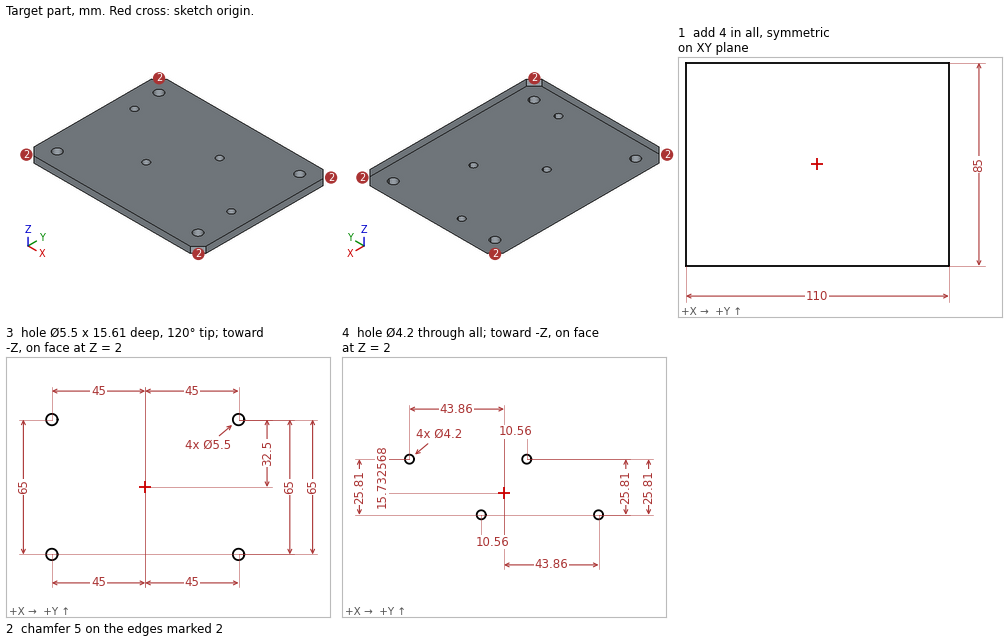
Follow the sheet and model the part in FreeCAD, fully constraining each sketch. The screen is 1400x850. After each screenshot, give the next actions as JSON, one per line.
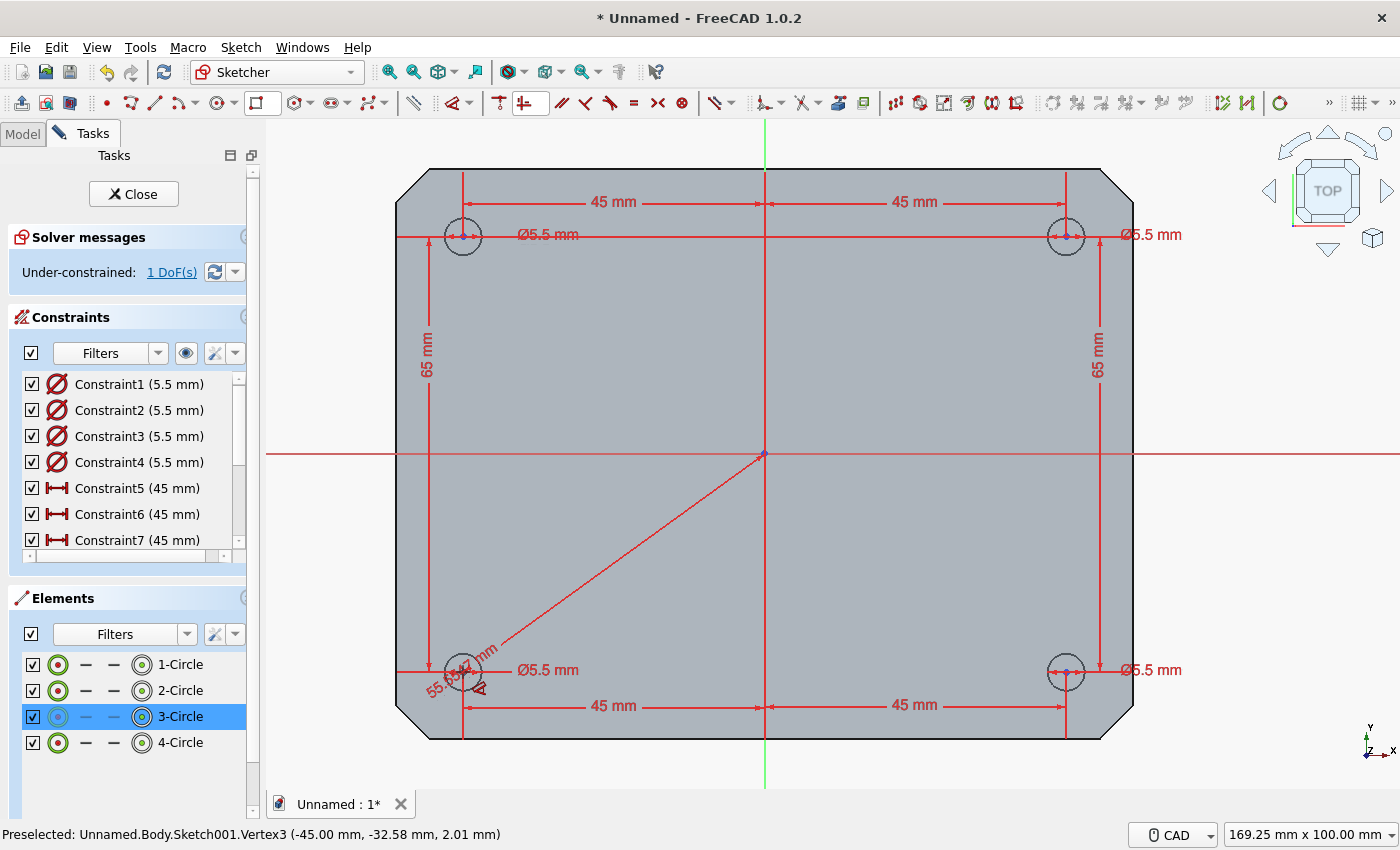
{"action": "left_click", "coordinate": [463, 237]}
{"action": "left_click", "coordinate": [429, 555]}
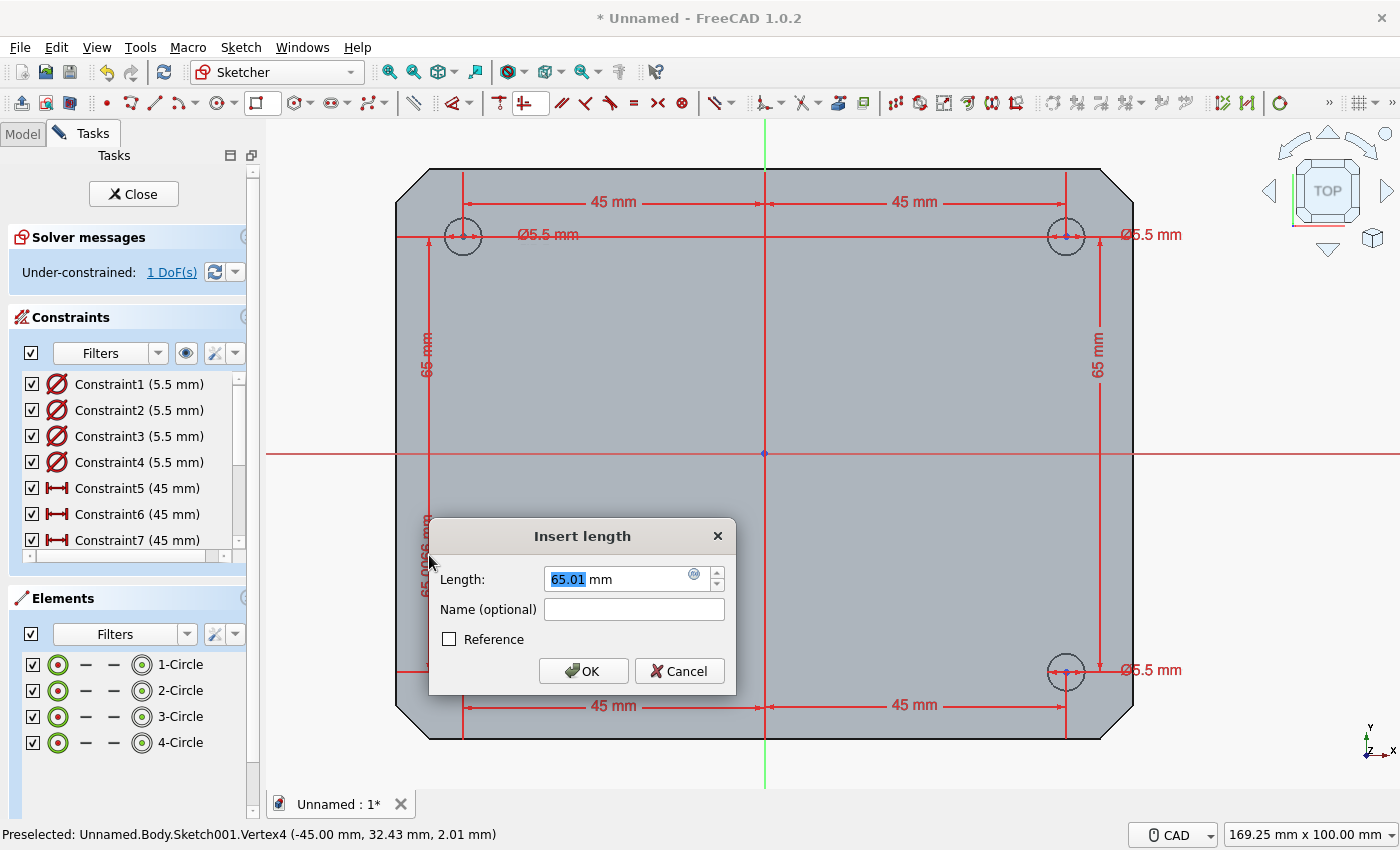
{"action": "type", "text": "65"}
{"action": "key", "text": "Return"}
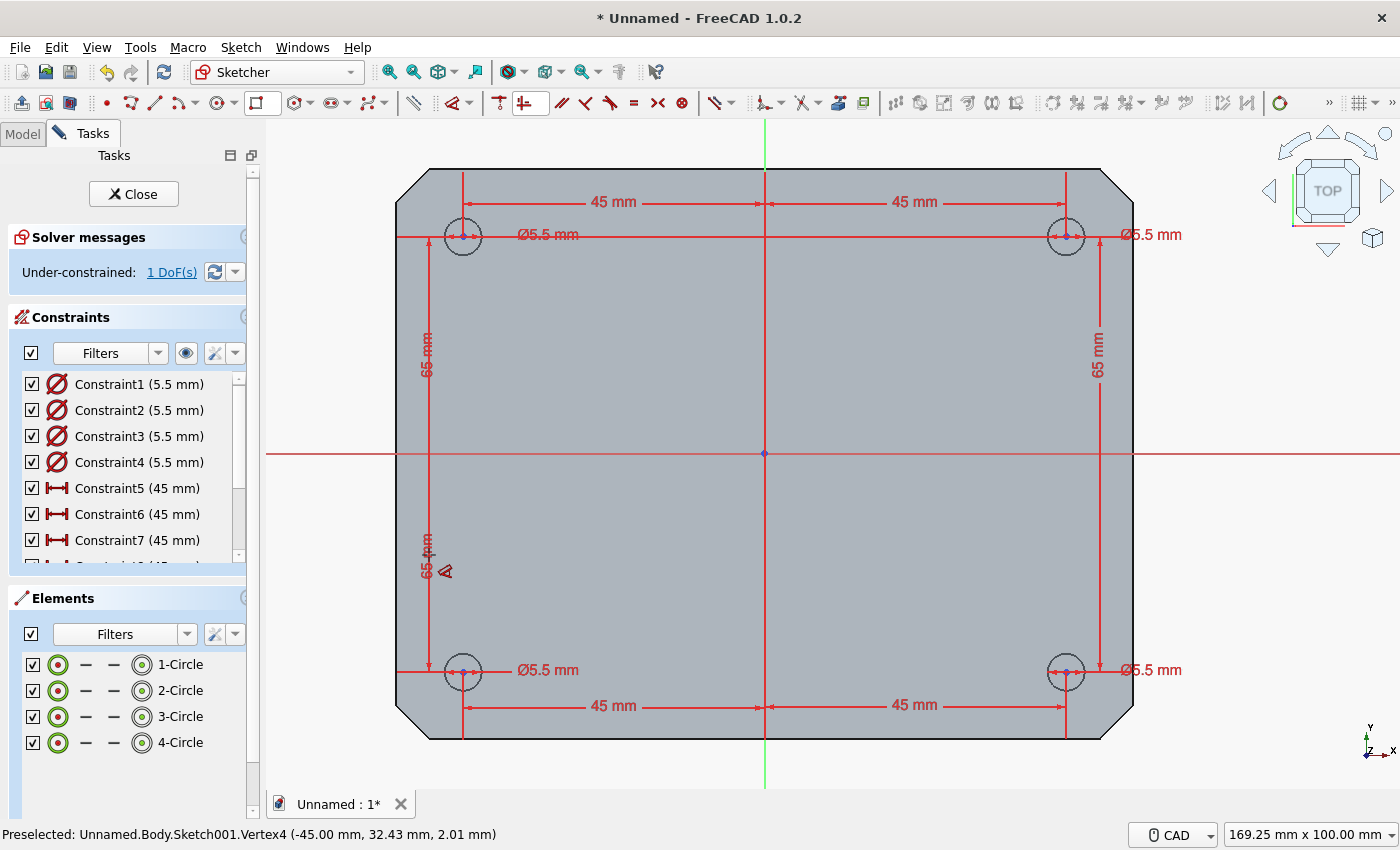
{"action": "left_click", "coordinate": [1066, 237]}
{"action": "left_click", "coordinate": [1100, 295]}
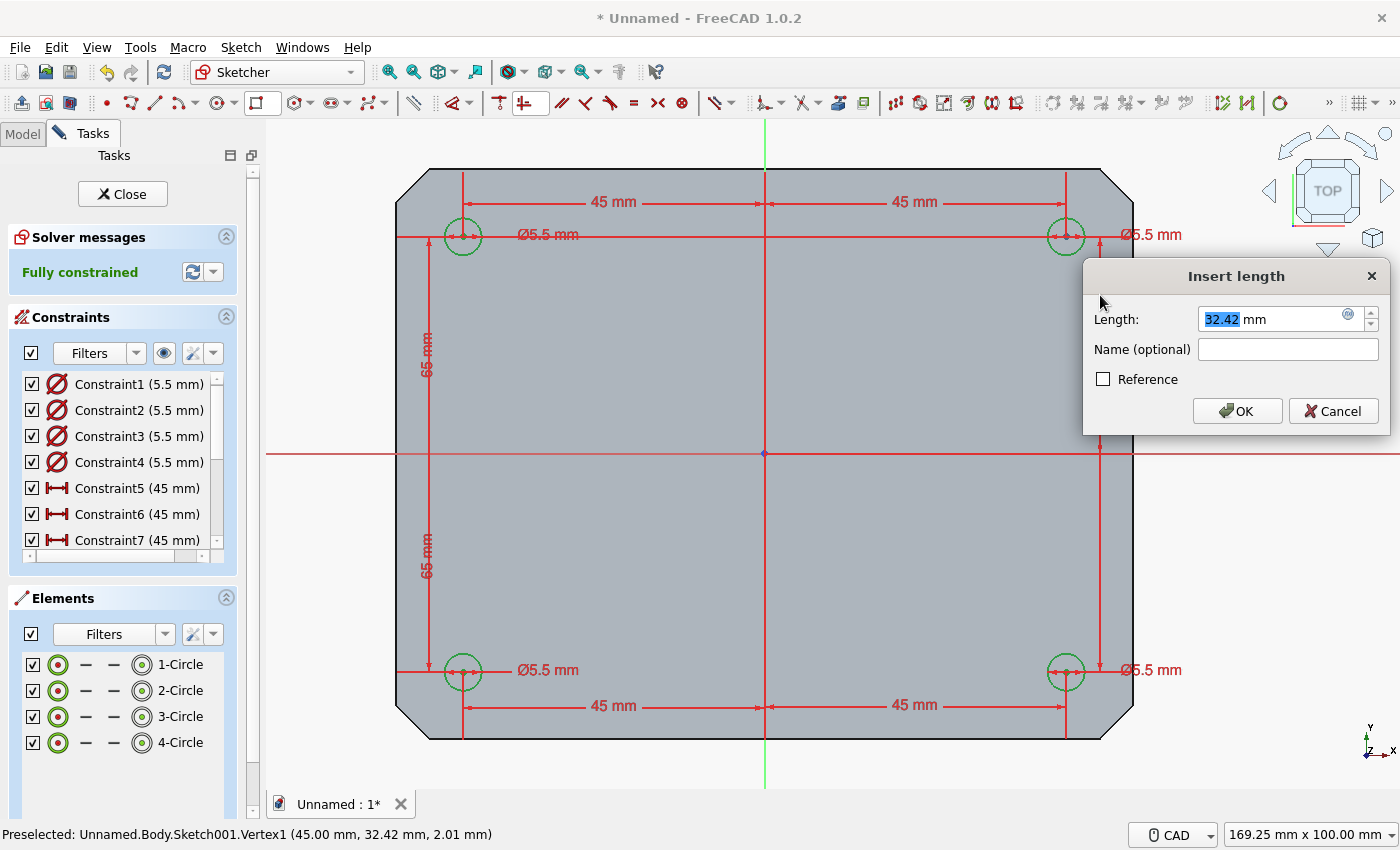
{"action": "type", "text": "32.5"}
{"action": "key", "text": "Return"}
{"action": "key", "text": "Escape"}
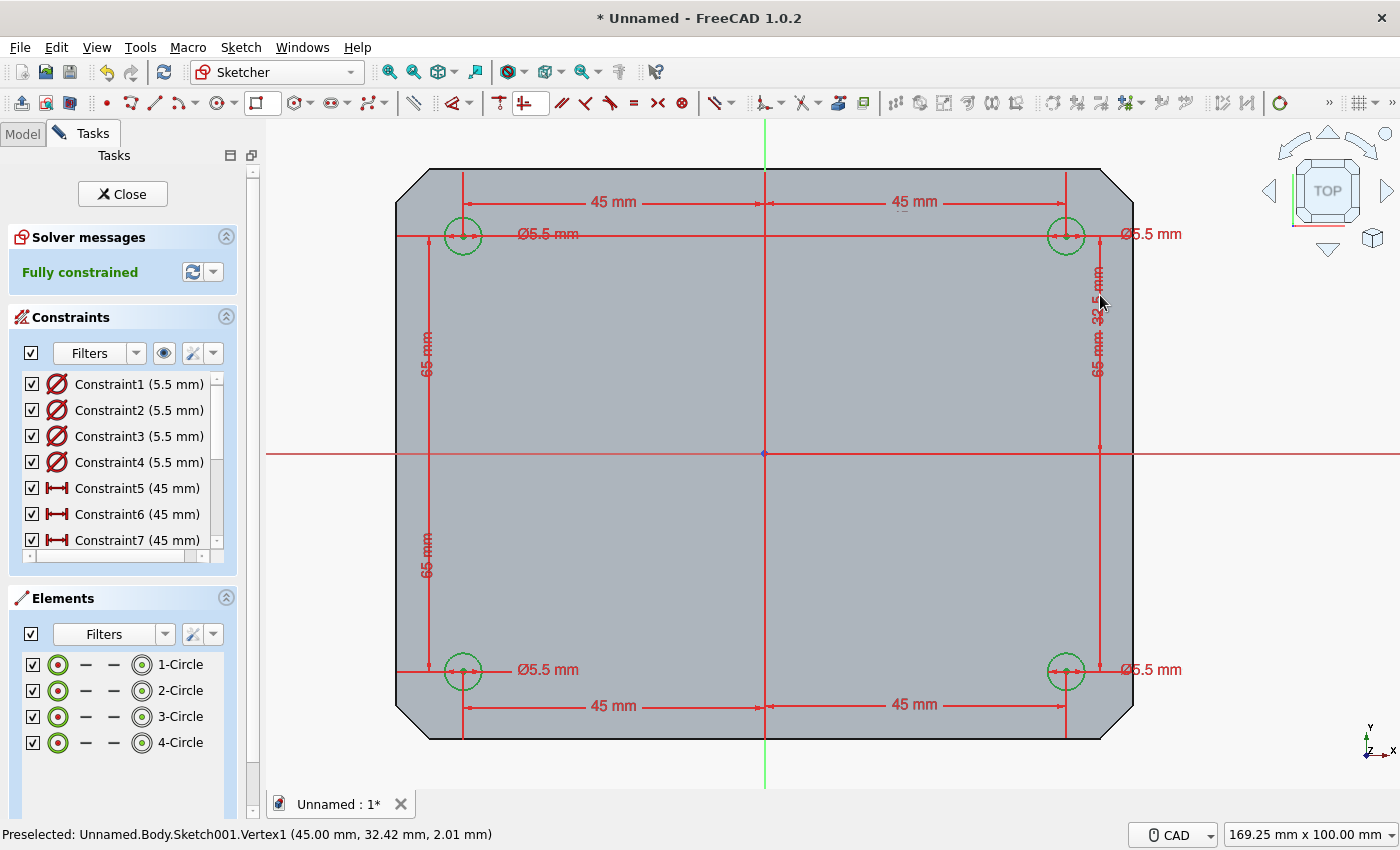
{"action": "left_click", "coordinate": [123, 194]}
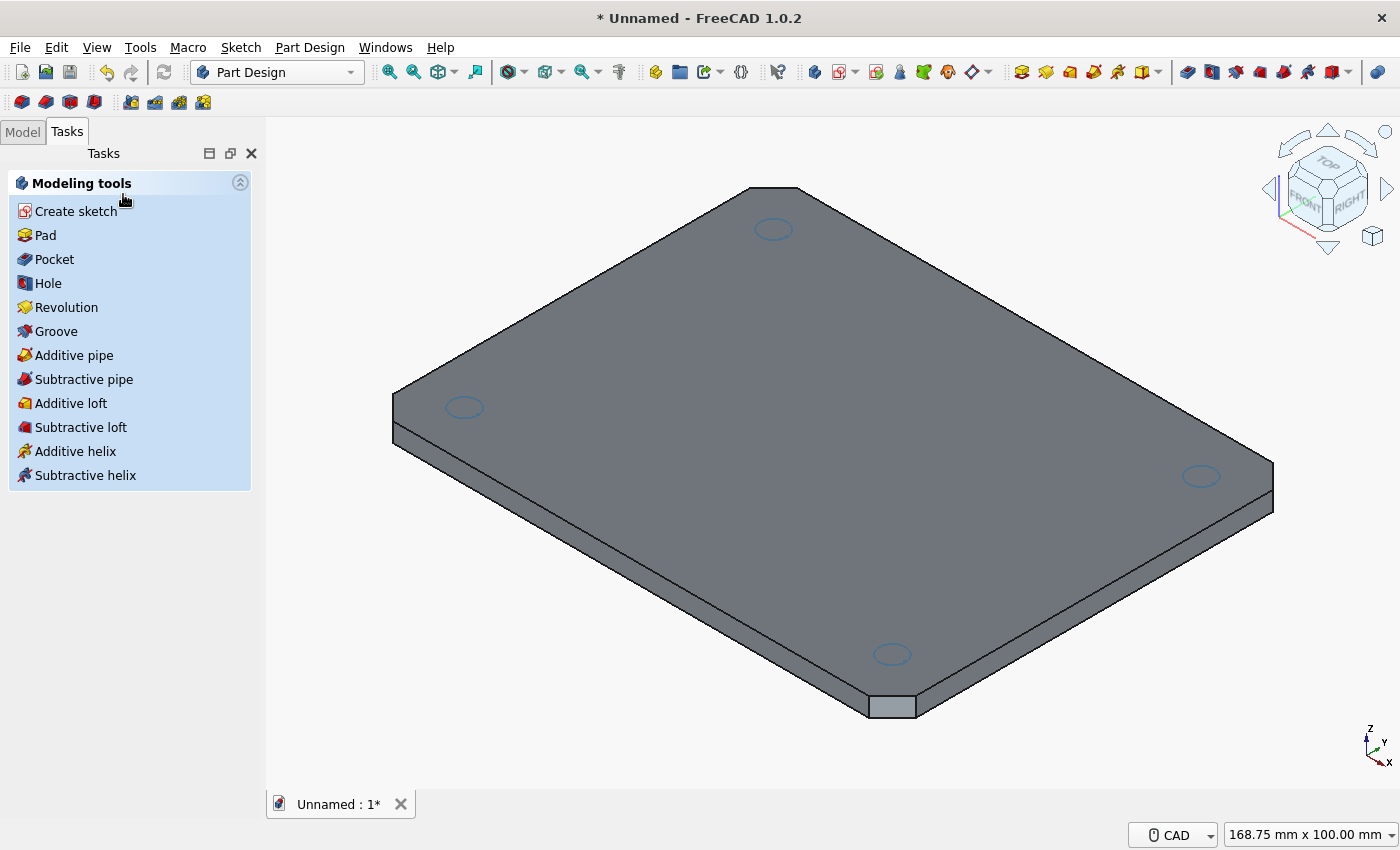
{"action": "left_click", "coordinate": [1212, 72]}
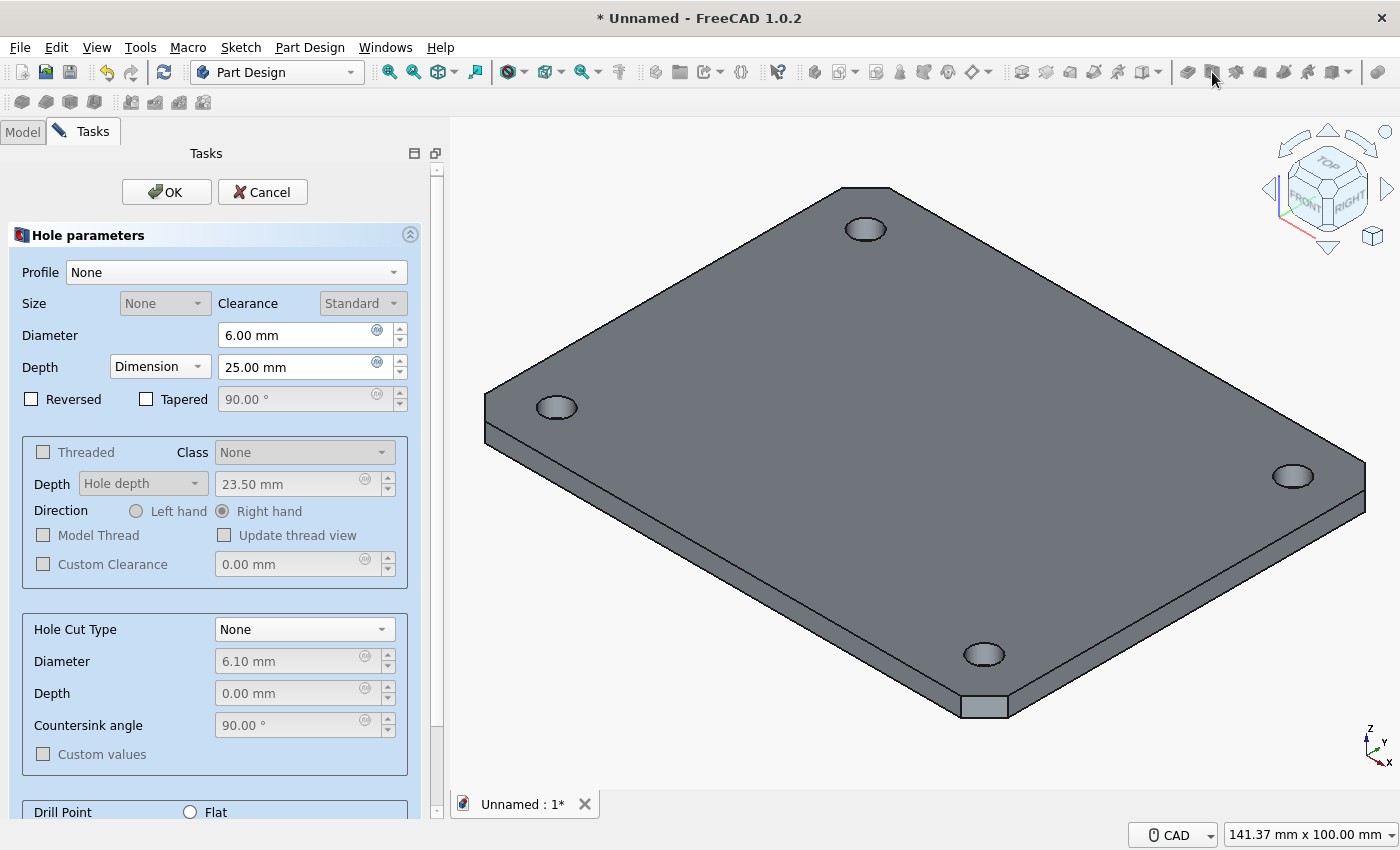
{"action": "triple_click", "coordinate": [305, 335]}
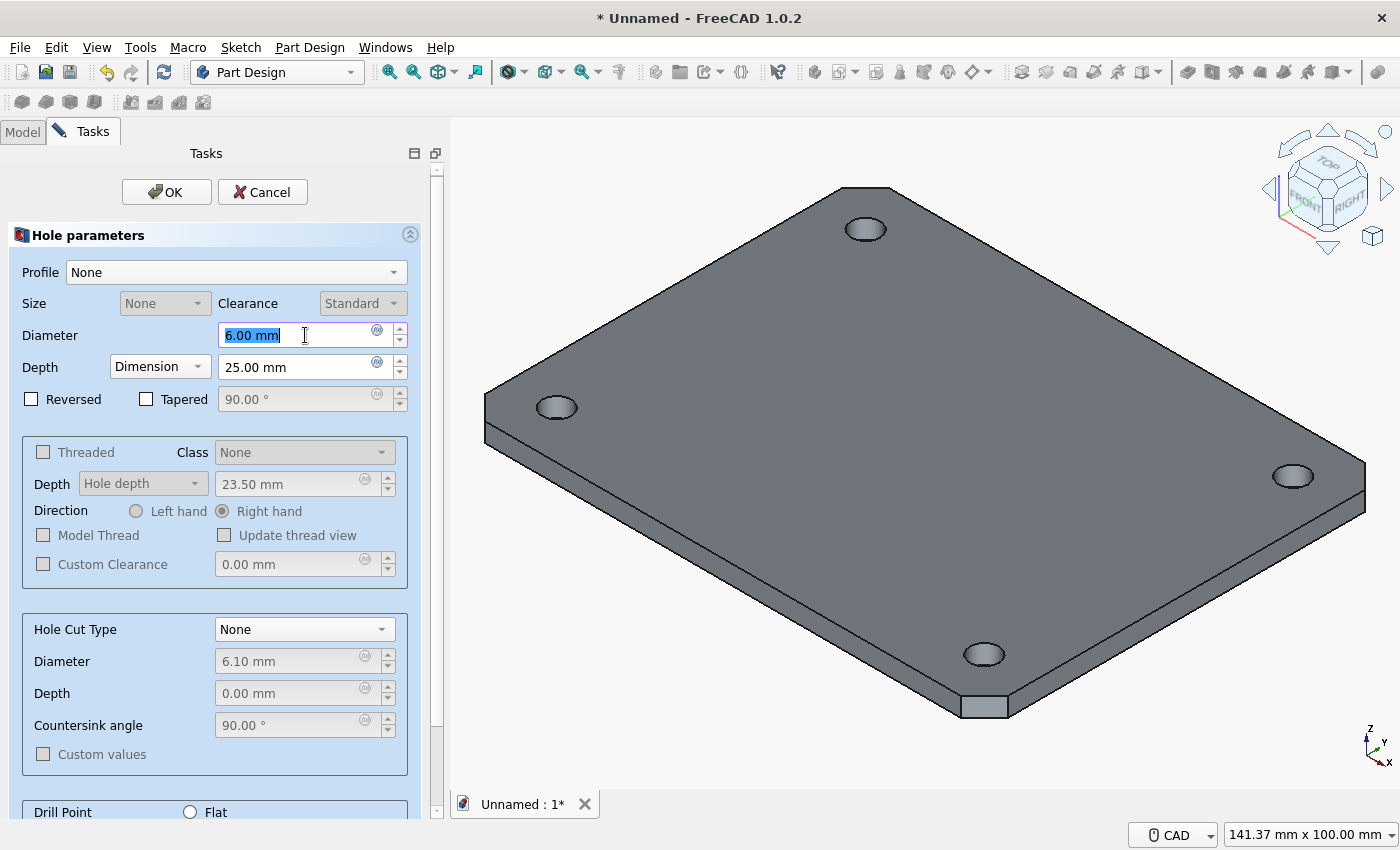
{"action": "type", "text": "5.5"}
{"action": "key", "text": "Tab"}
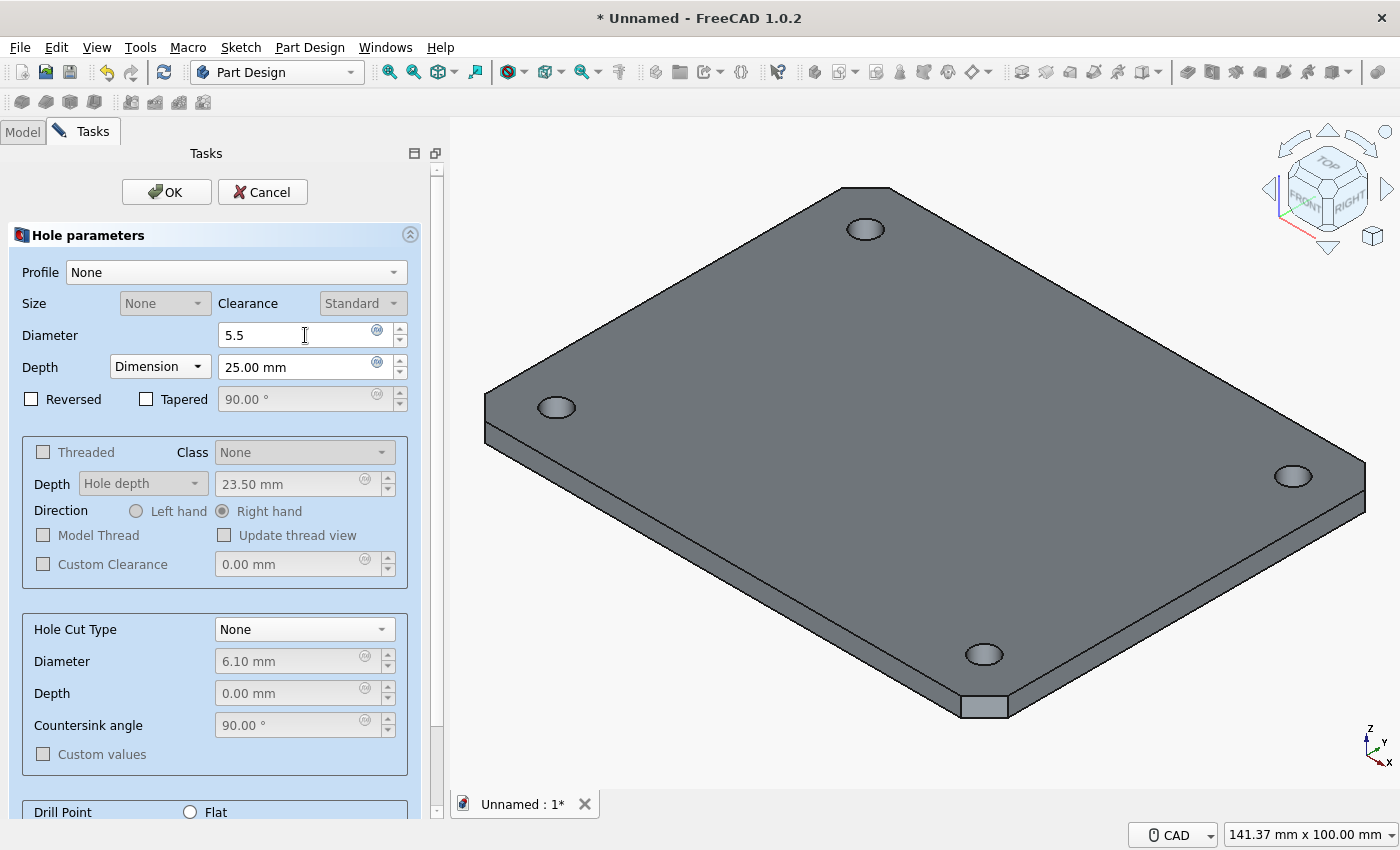
{"action": "triple_click", "coordinate": [305, 367]}